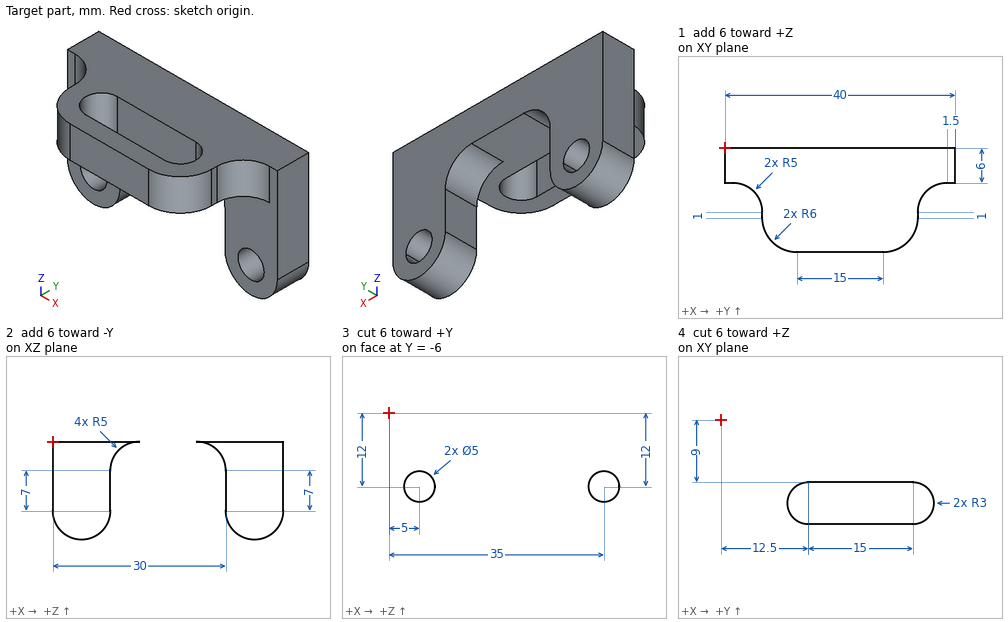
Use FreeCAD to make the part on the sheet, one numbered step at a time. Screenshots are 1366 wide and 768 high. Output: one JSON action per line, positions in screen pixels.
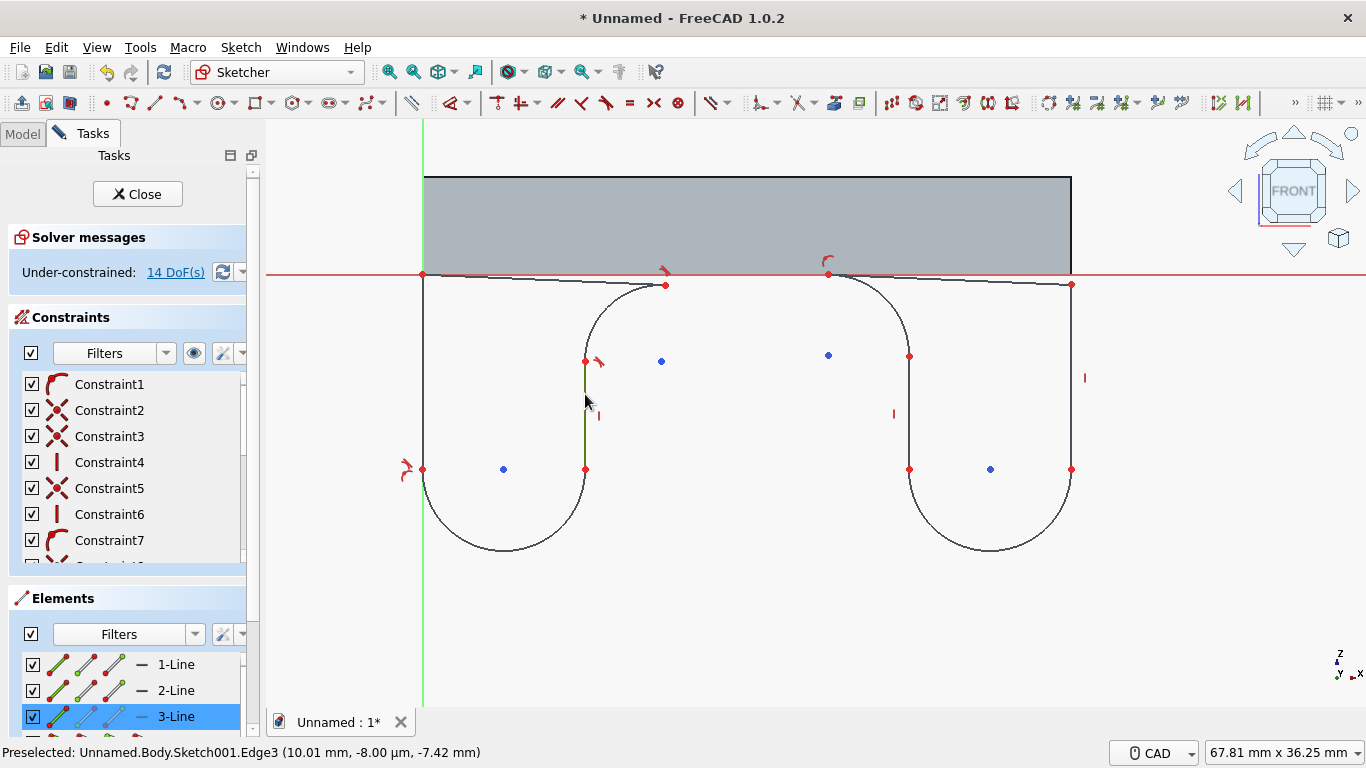
{"action": "left_click", "coordinate": [456, 535]}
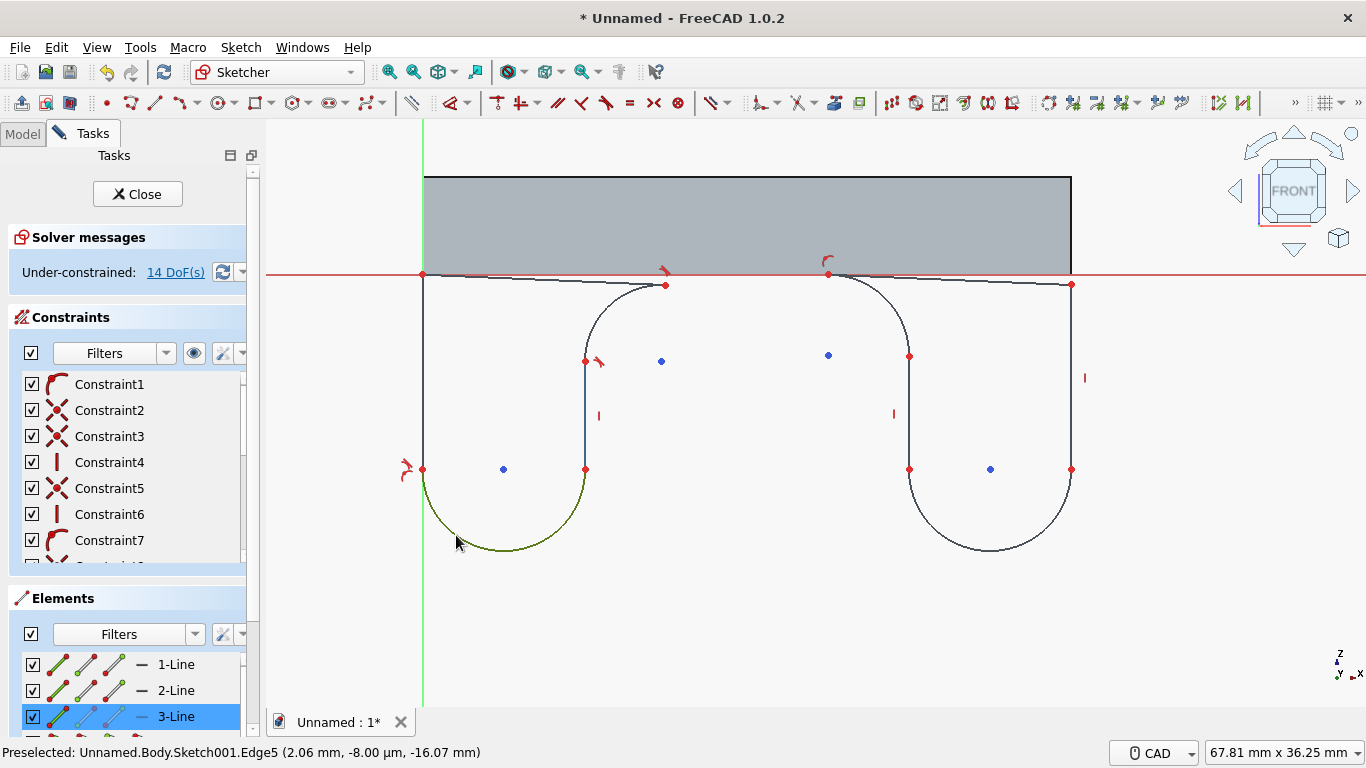
{"action": "key", "text": "t"}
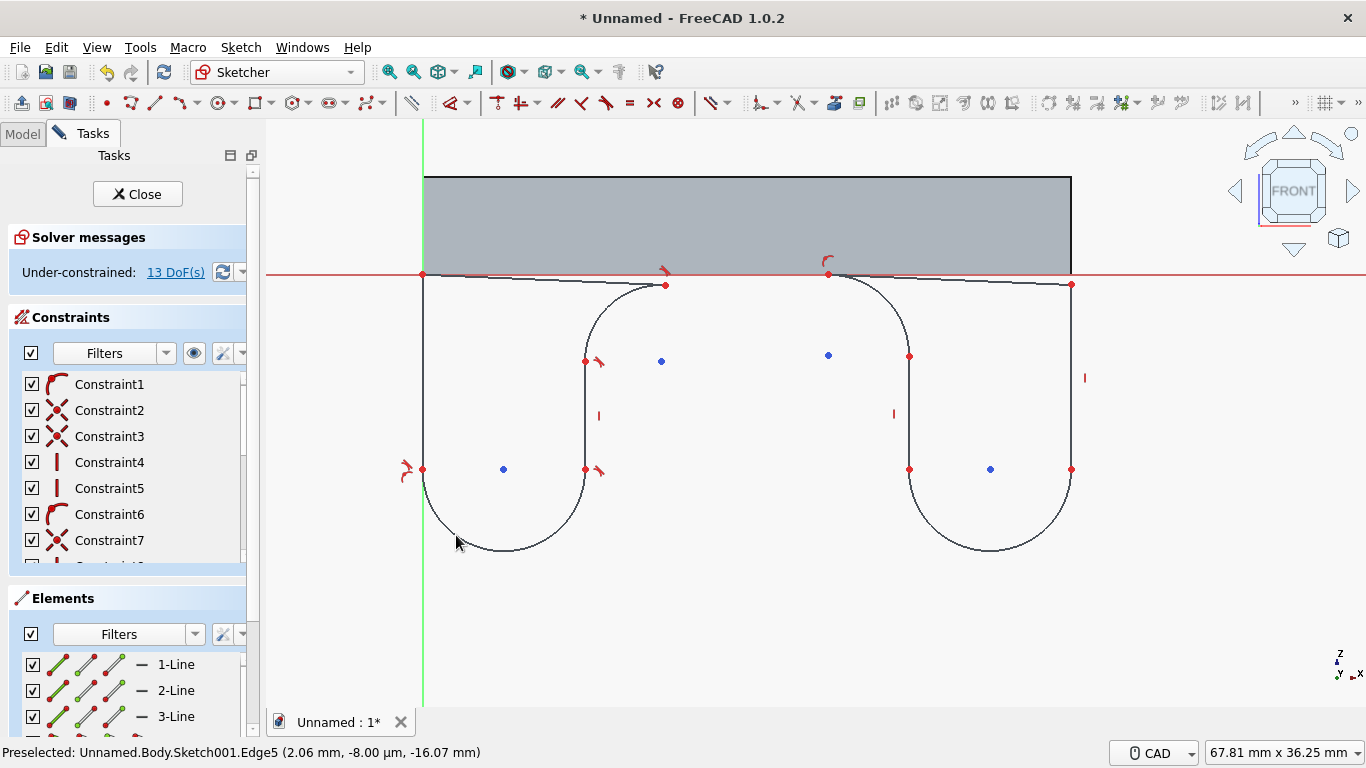
{"action": "left_click", "coordinate": [909, 436]}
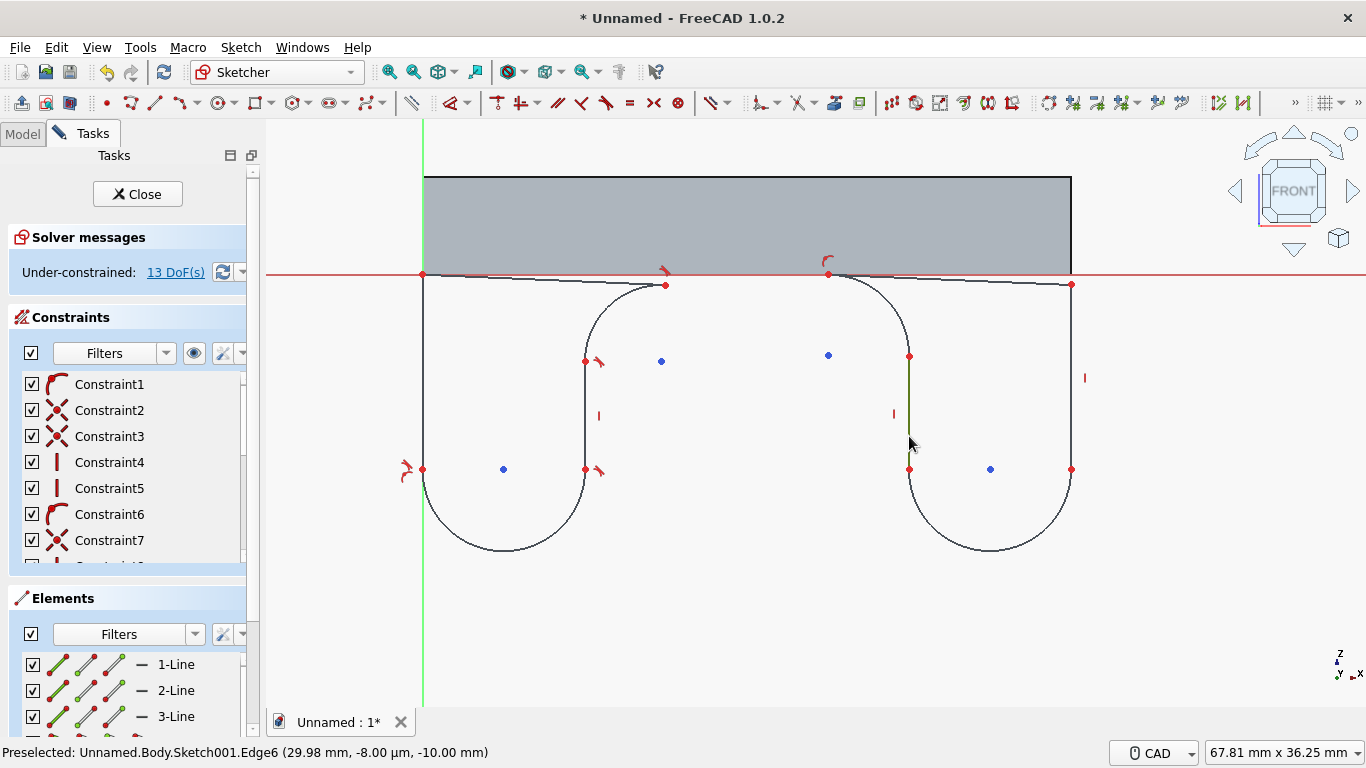
{"action": "left_click", "coordinate": [901, 320]}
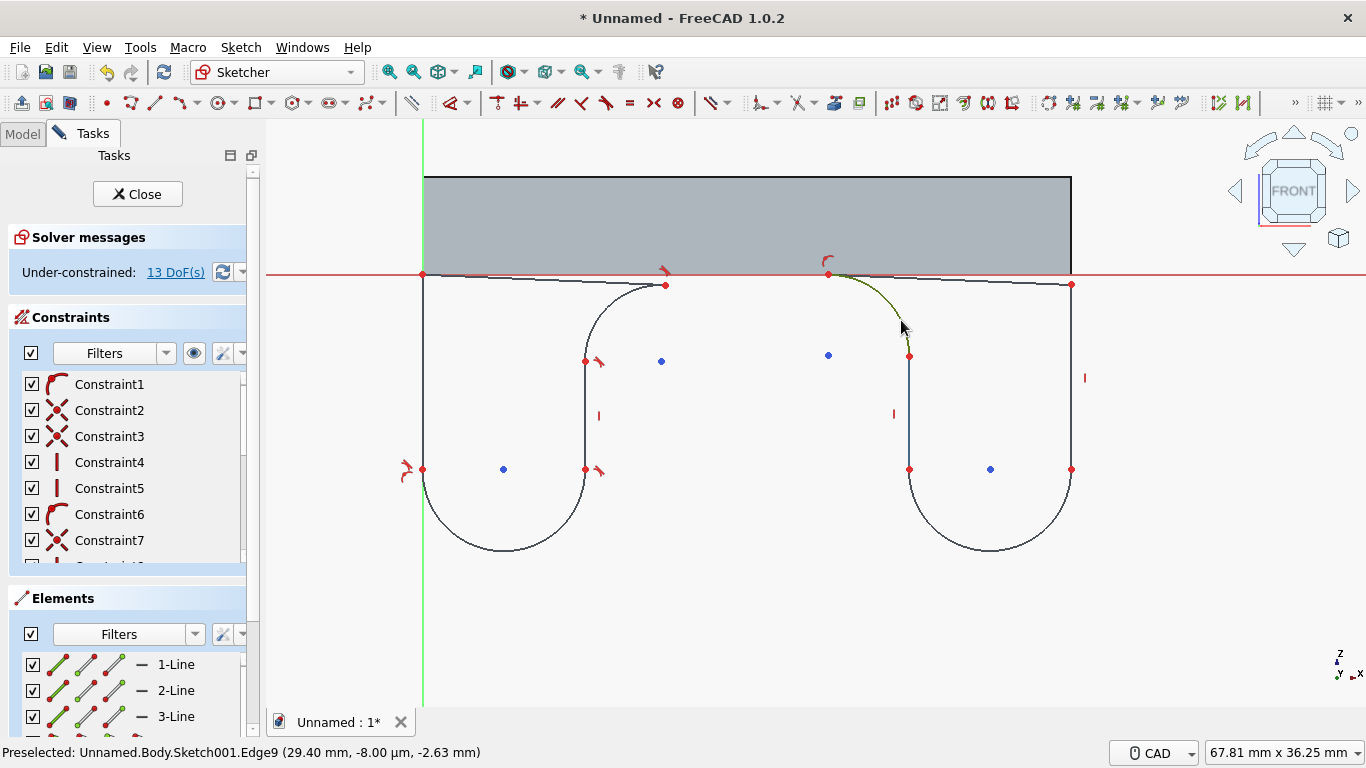
{"action": "left_click", "coordinate": [606, 104]}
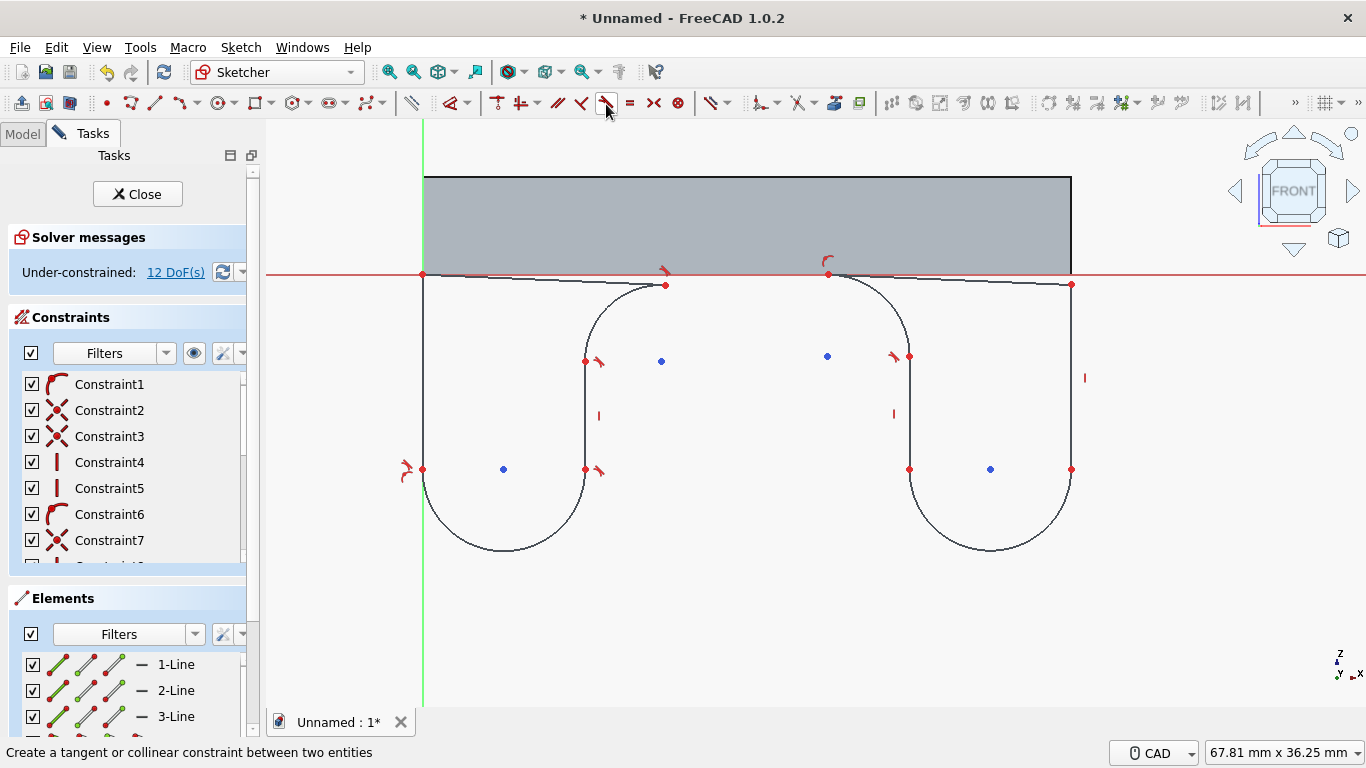
{"action": "left_click", "coordinate": [910, 436]}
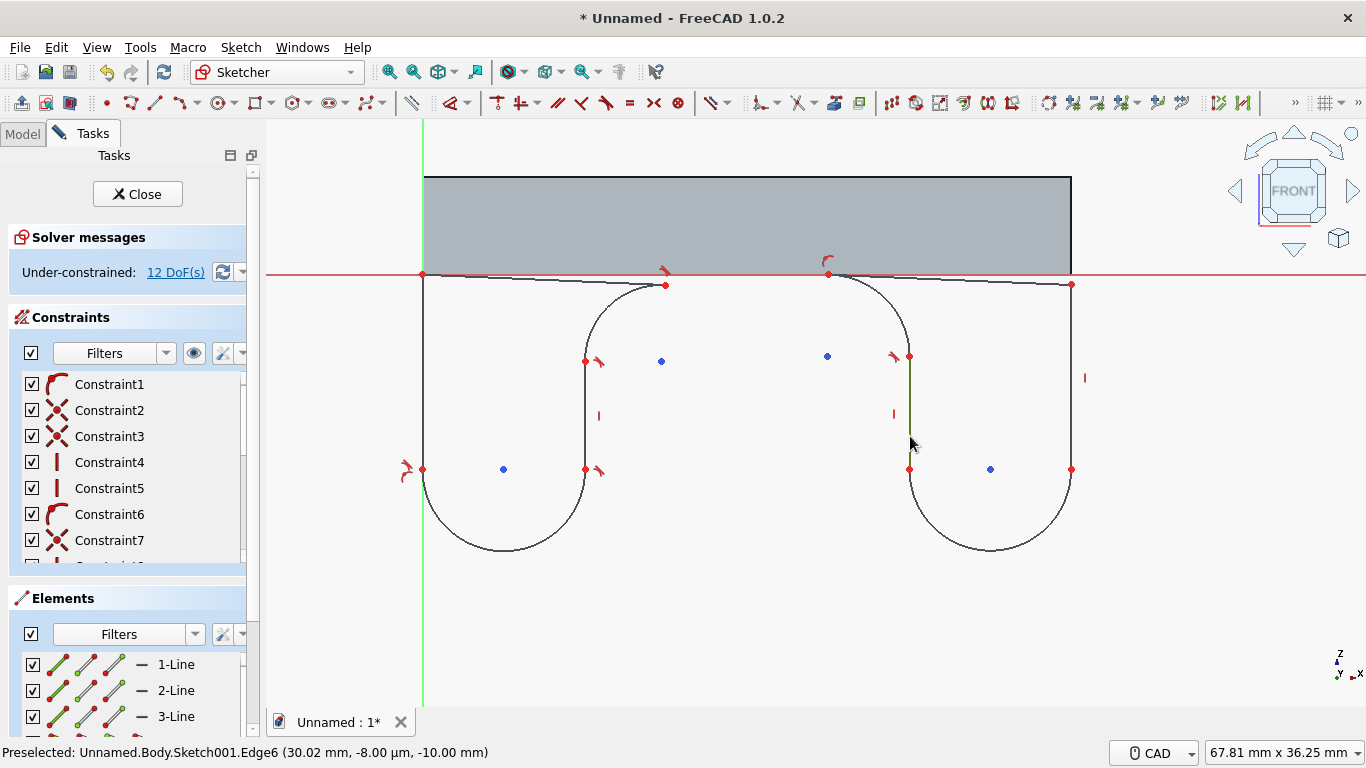
{"action": "left_click", "coordinate": [943, 535]}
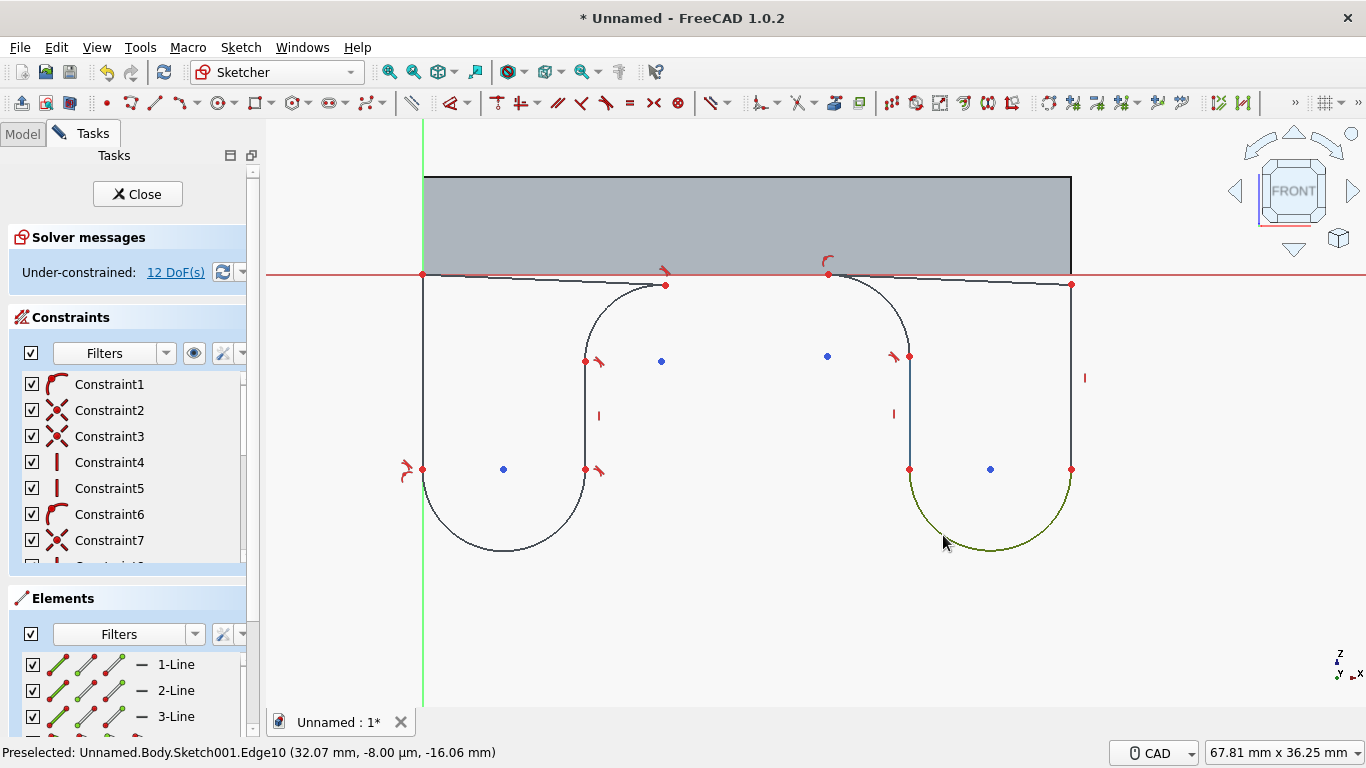
{"action": "left_click", "coordinate": [606, 104]}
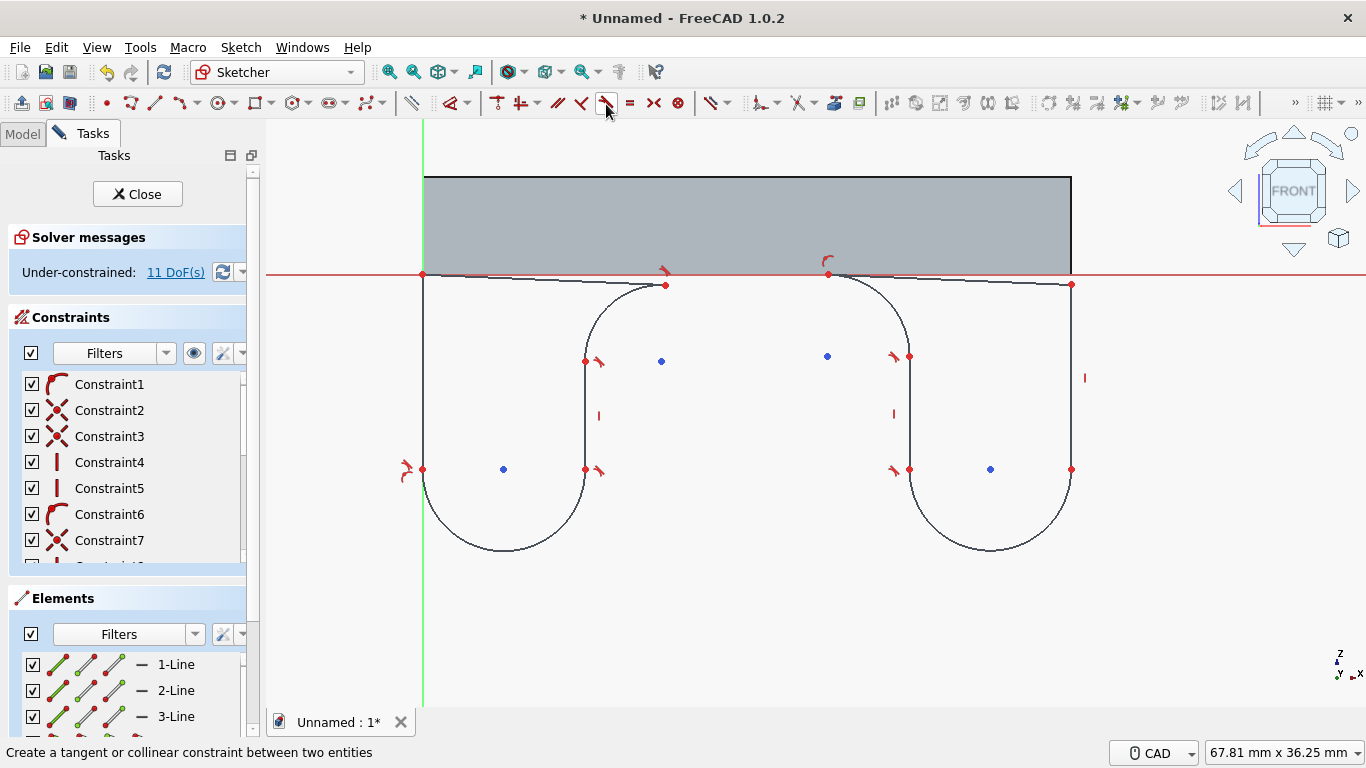
{"action": "left_click", "coordinate": [901, 278]}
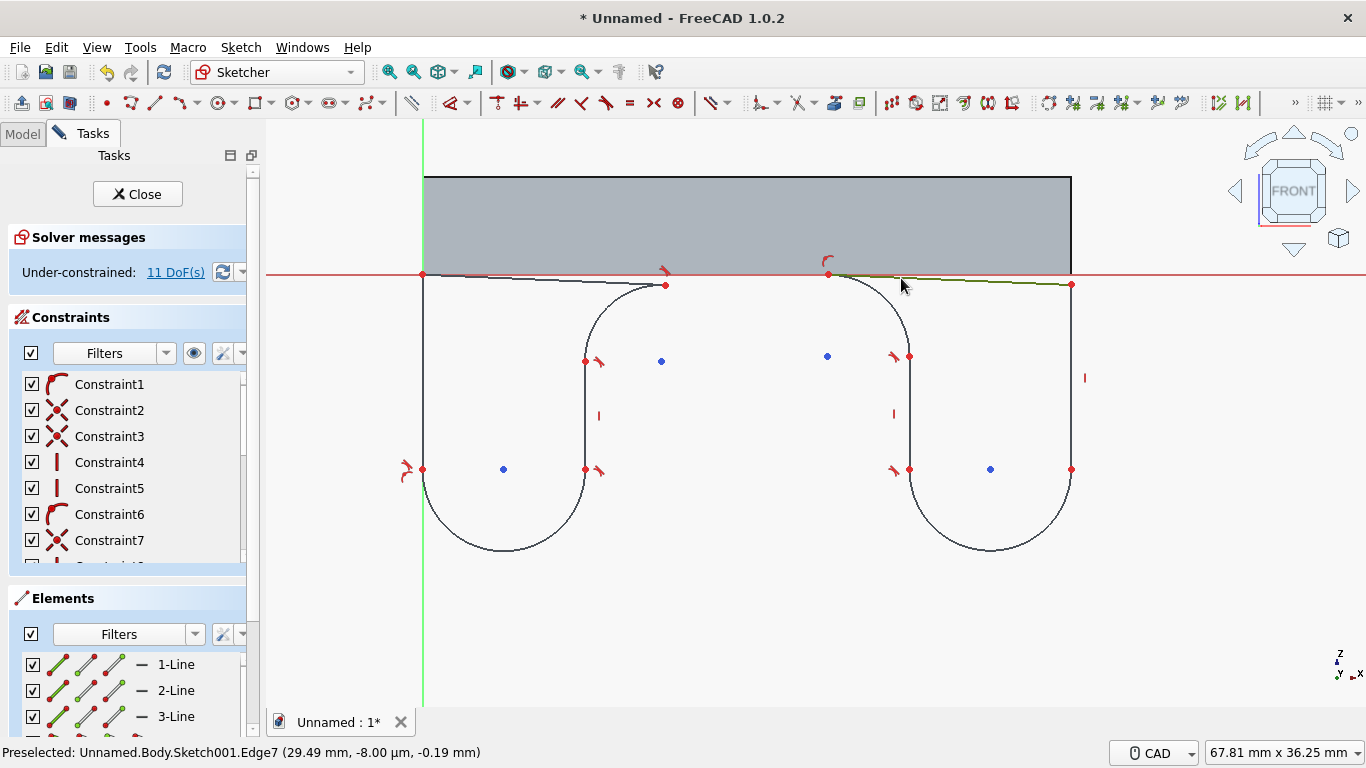
{"action": "left_click", "coordinate": [901, 320]}